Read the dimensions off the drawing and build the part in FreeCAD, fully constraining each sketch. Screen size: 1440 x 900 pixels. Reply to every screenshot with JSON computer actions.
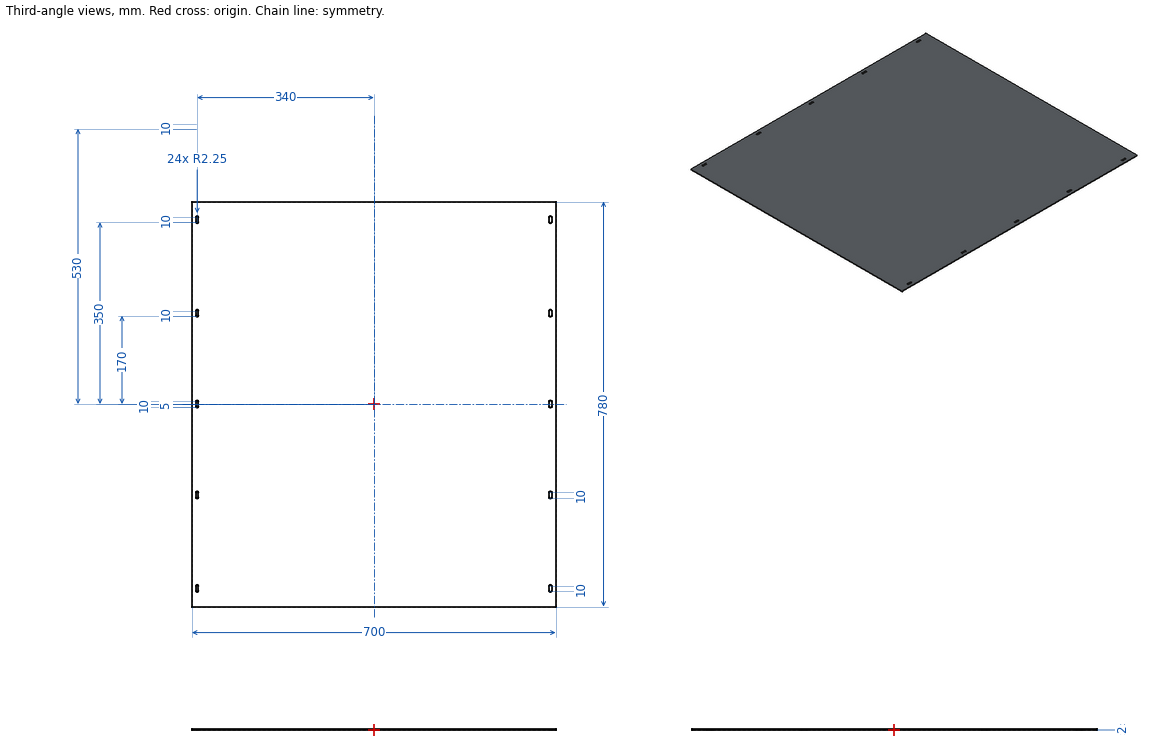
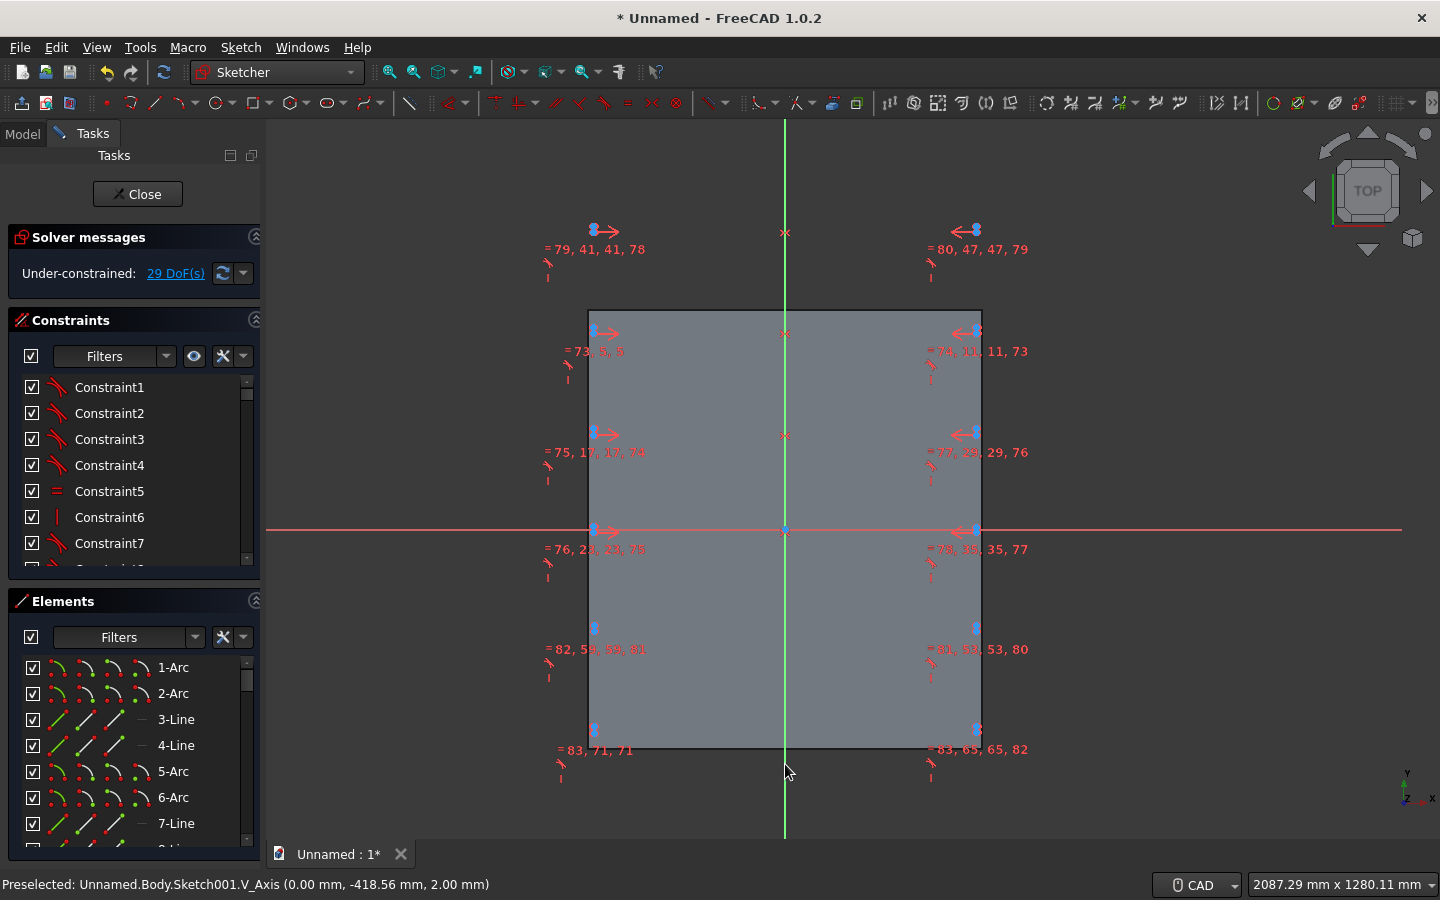
{"action": "scroll", "coordinate": [977, 429], "scroll_direction": "up", "scroll_amount": 12}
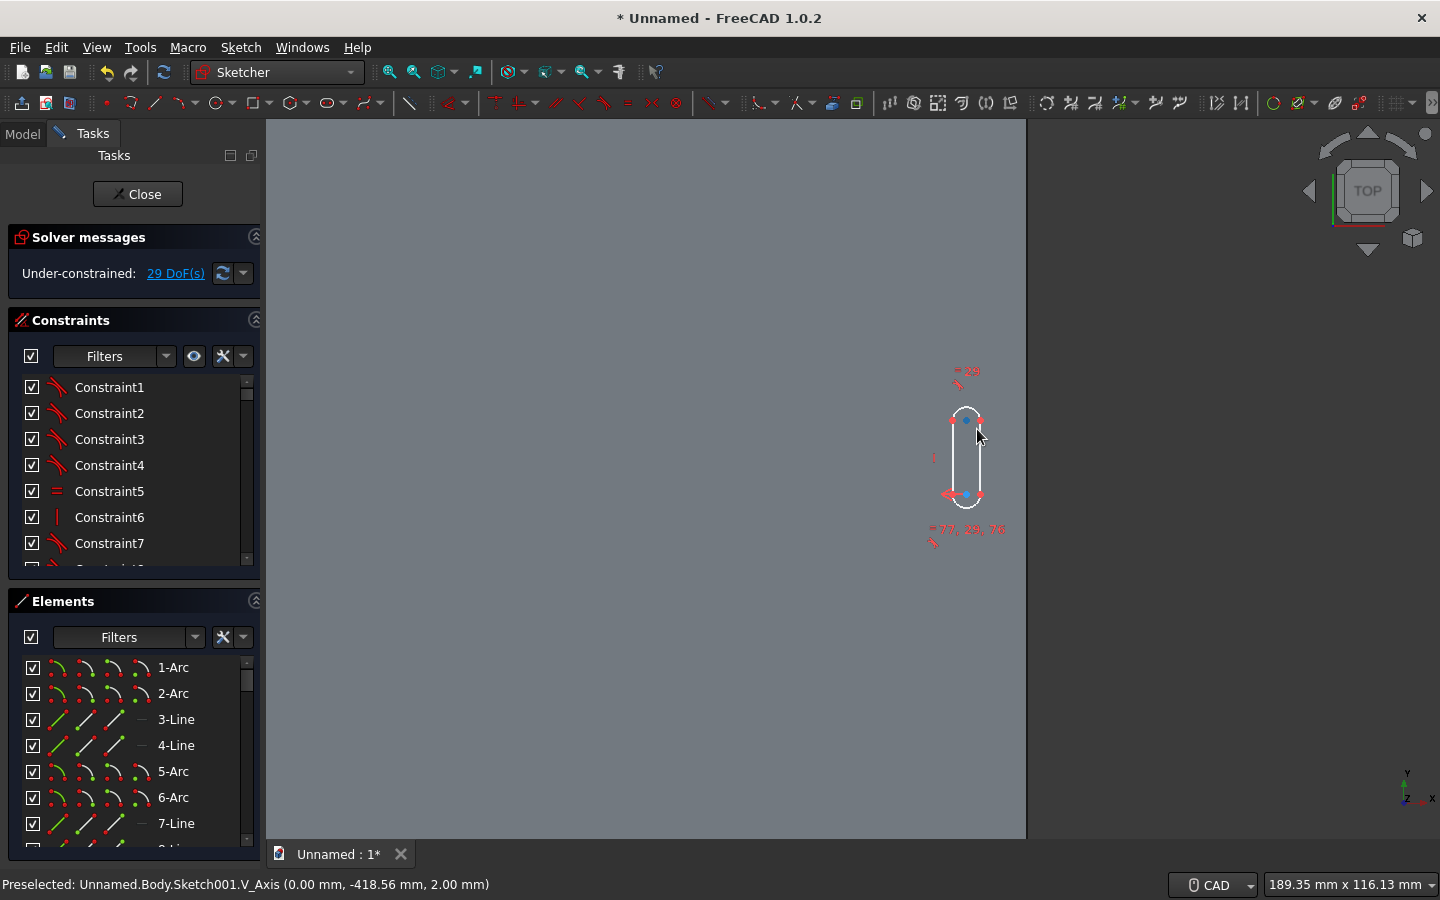
{"action": "left_click", "coordinate": [966, 421]}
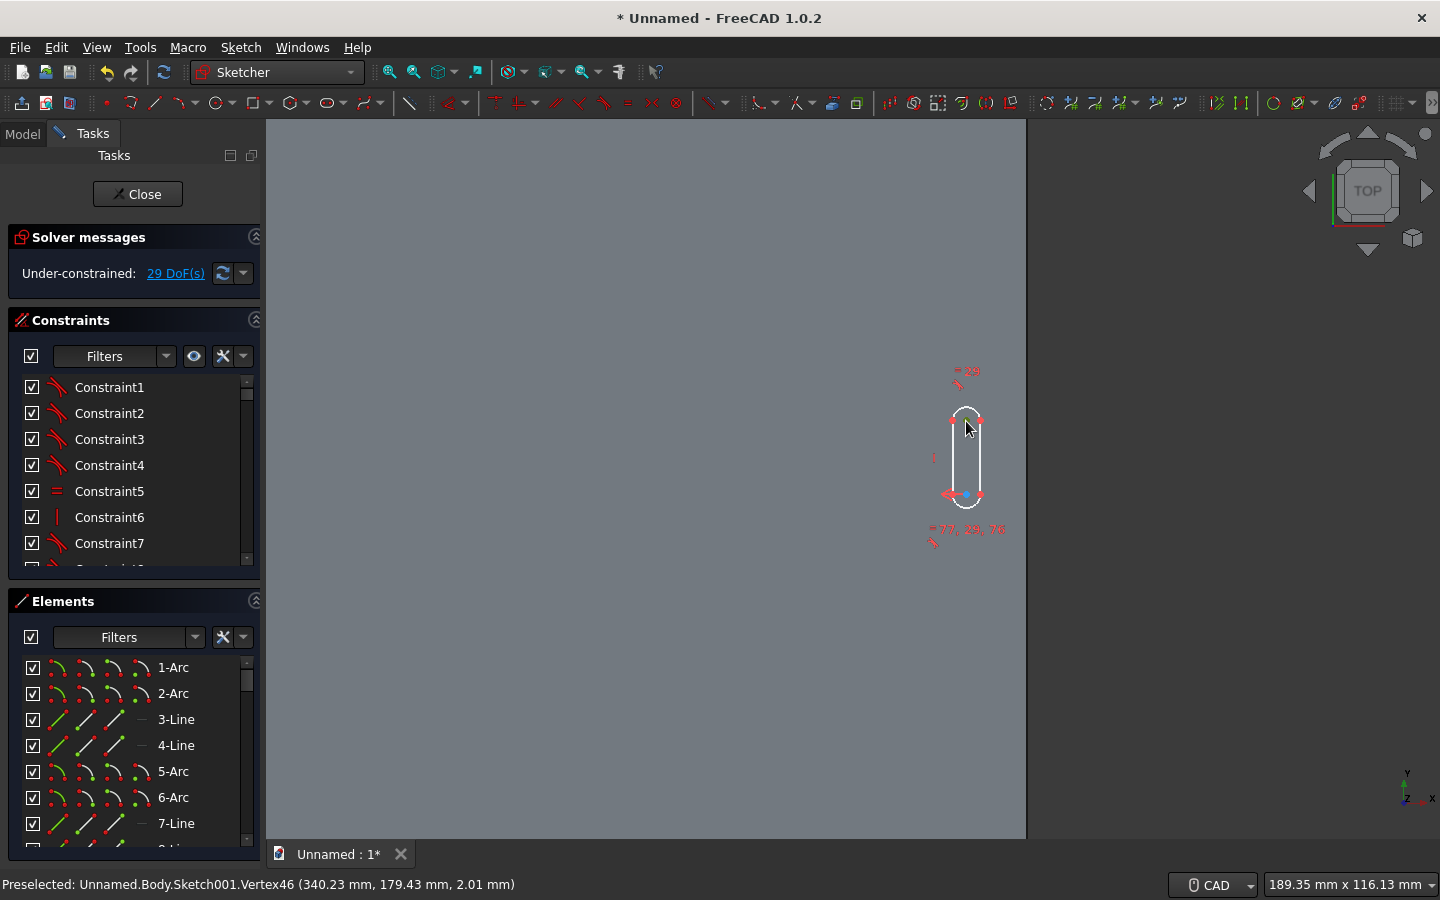
{"action": "scroll", "coordinate": [977, 429], "scroll_direction": "down", "scroll_amount": 12}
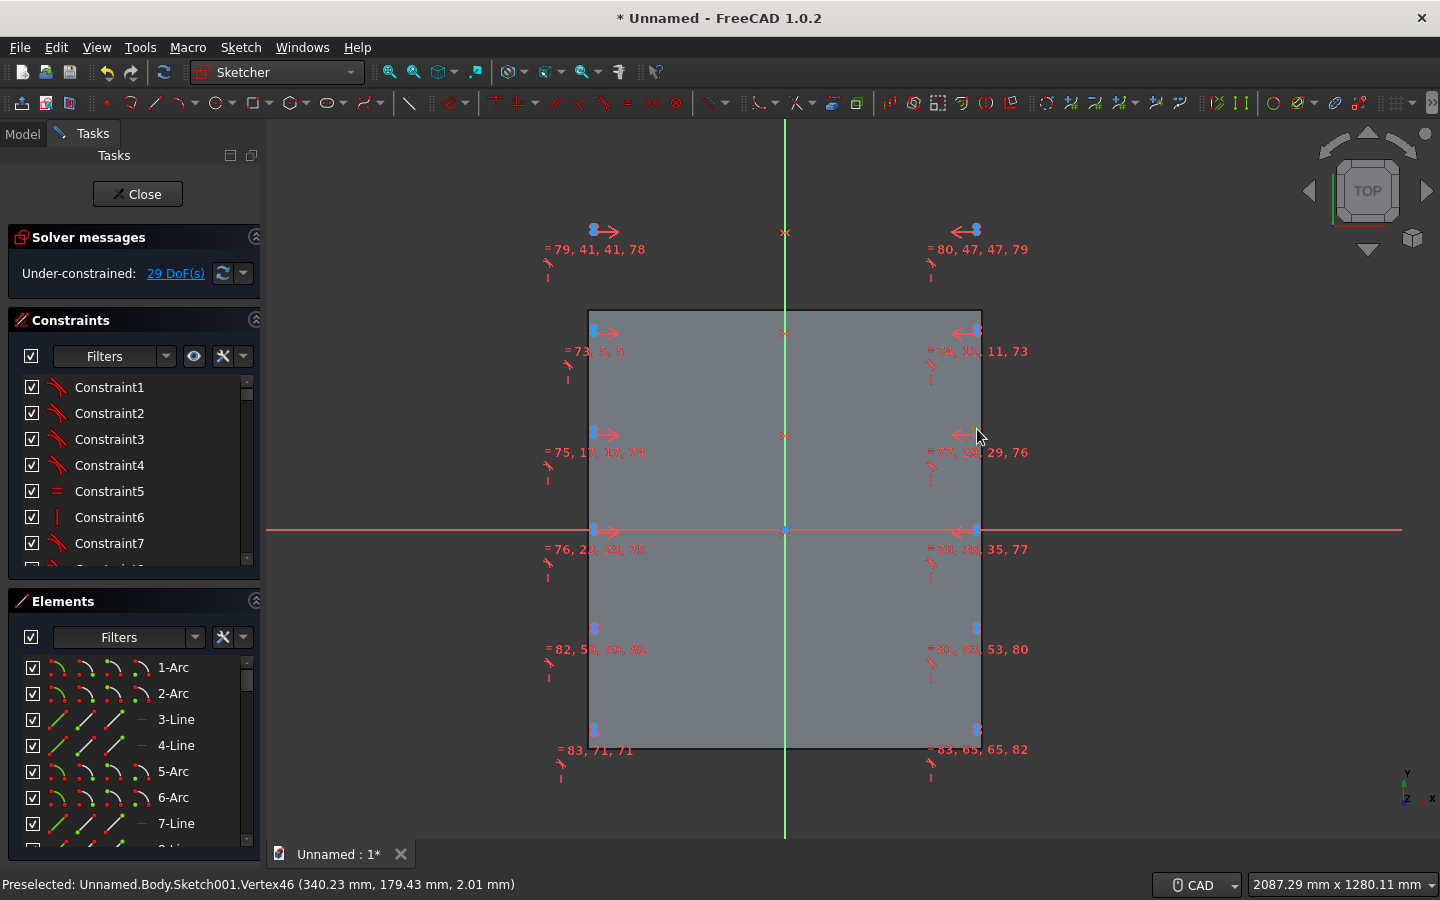
{"action": "scroll", "coordinate": [976, 632], "scroll_direction": "up", "scroll_amount": 12}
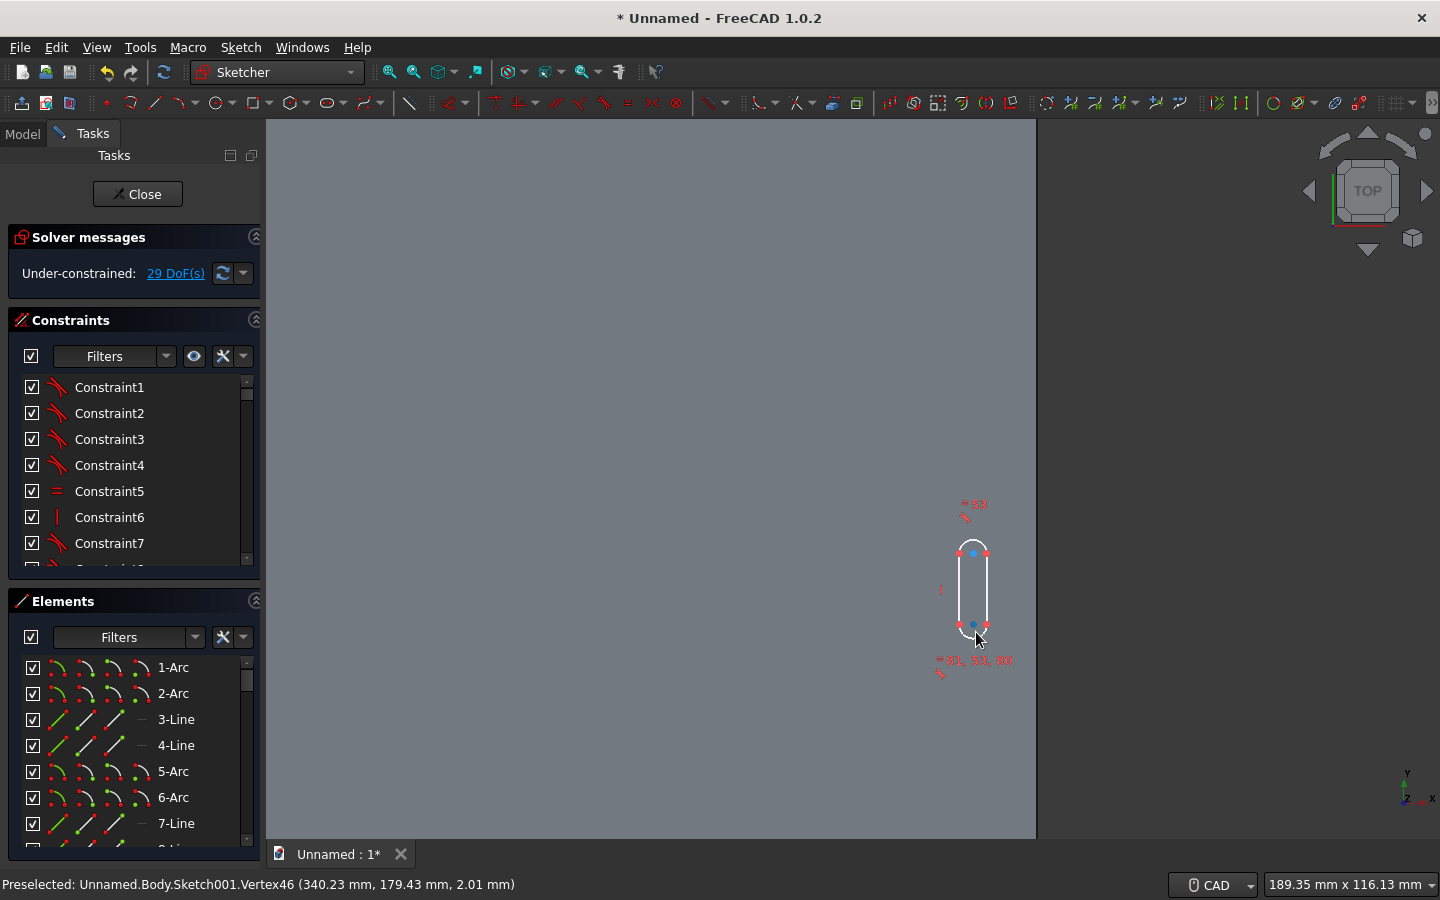
{"action": "left_click", "coordinate": [973, 625]}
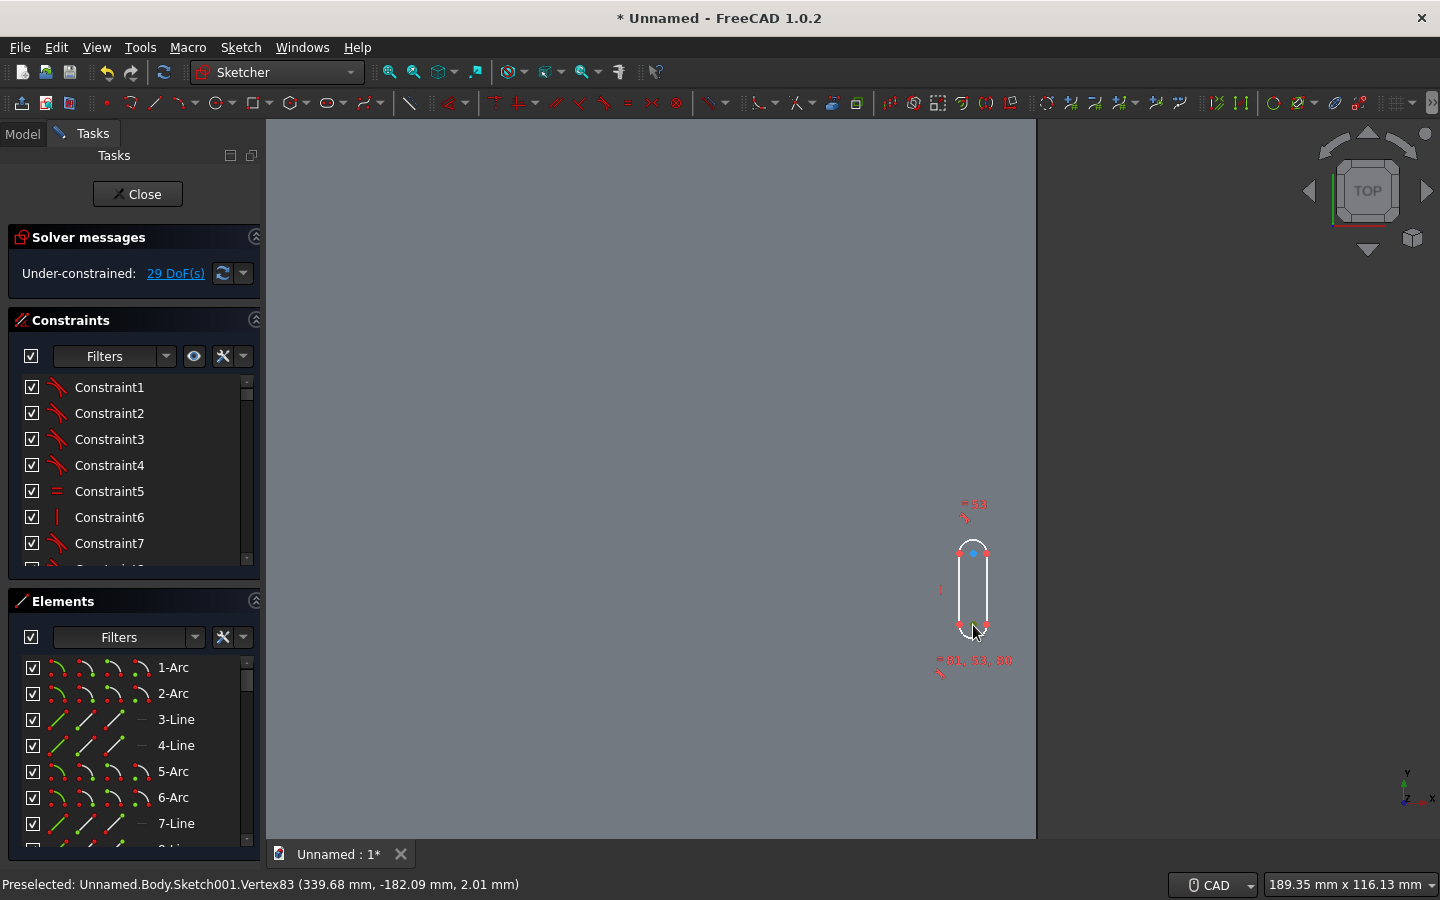
{"action": "scroll", "coordinate": [976, 633], "scroll_direction": "down", "scroll_amount": 12}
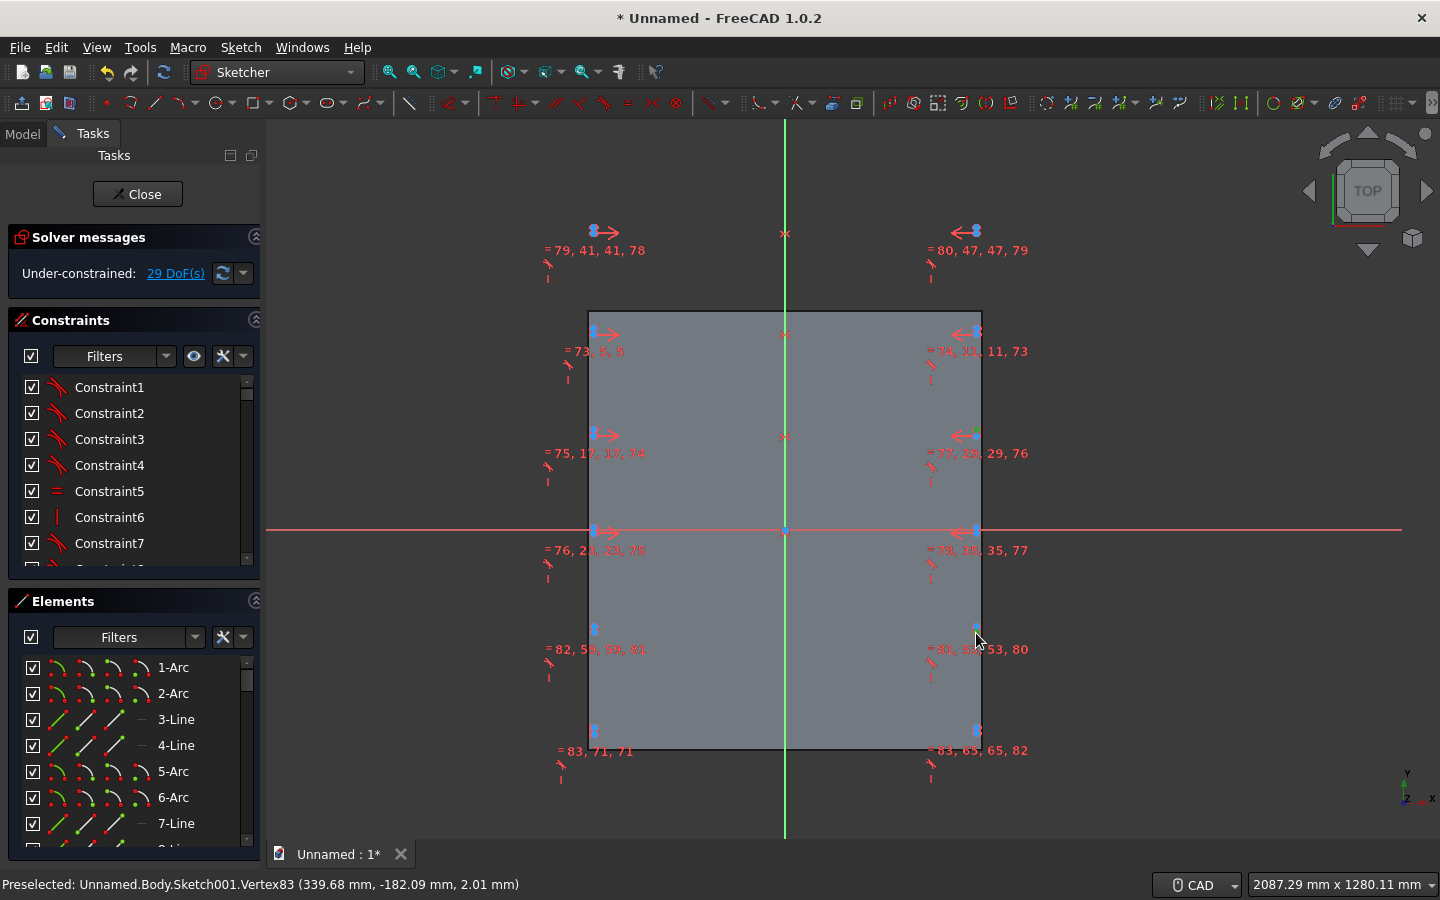
{"action": "left_click", "coordinate": [364, 530]}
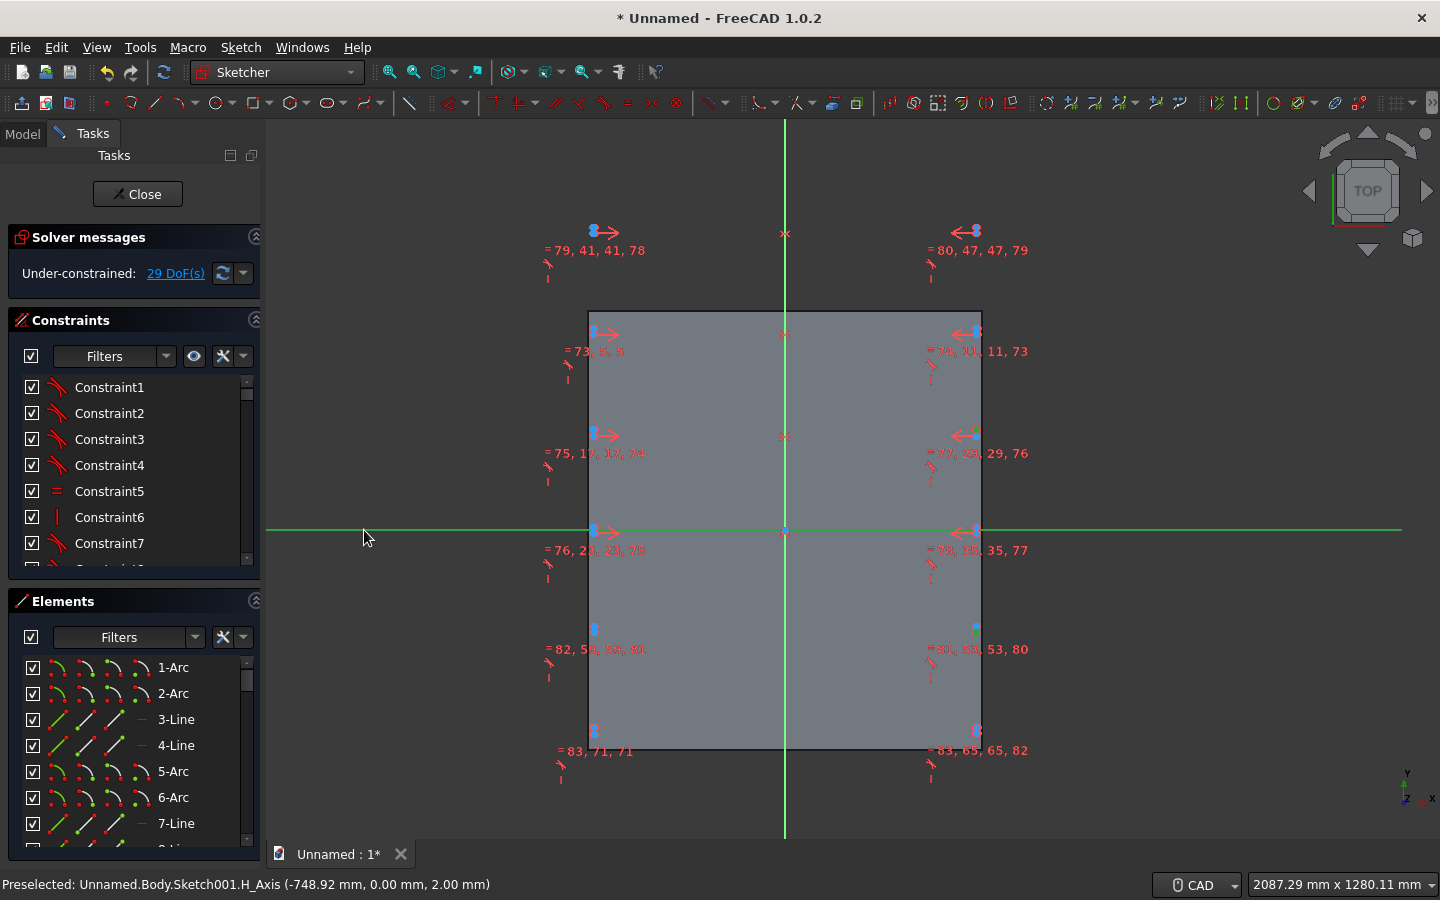
{"action": "key", "text": "s"}